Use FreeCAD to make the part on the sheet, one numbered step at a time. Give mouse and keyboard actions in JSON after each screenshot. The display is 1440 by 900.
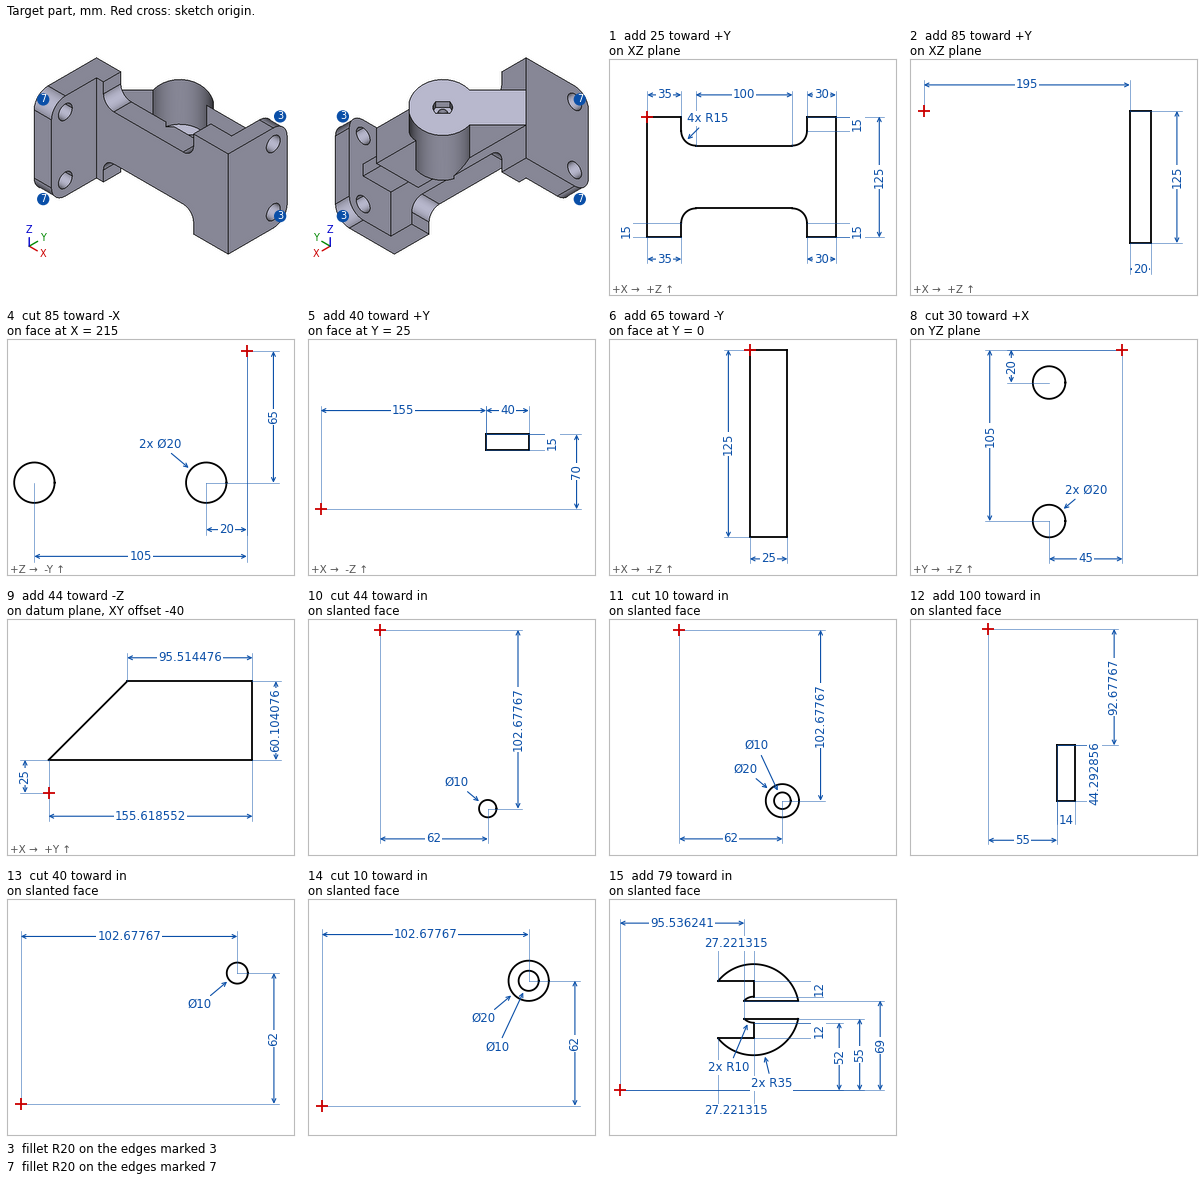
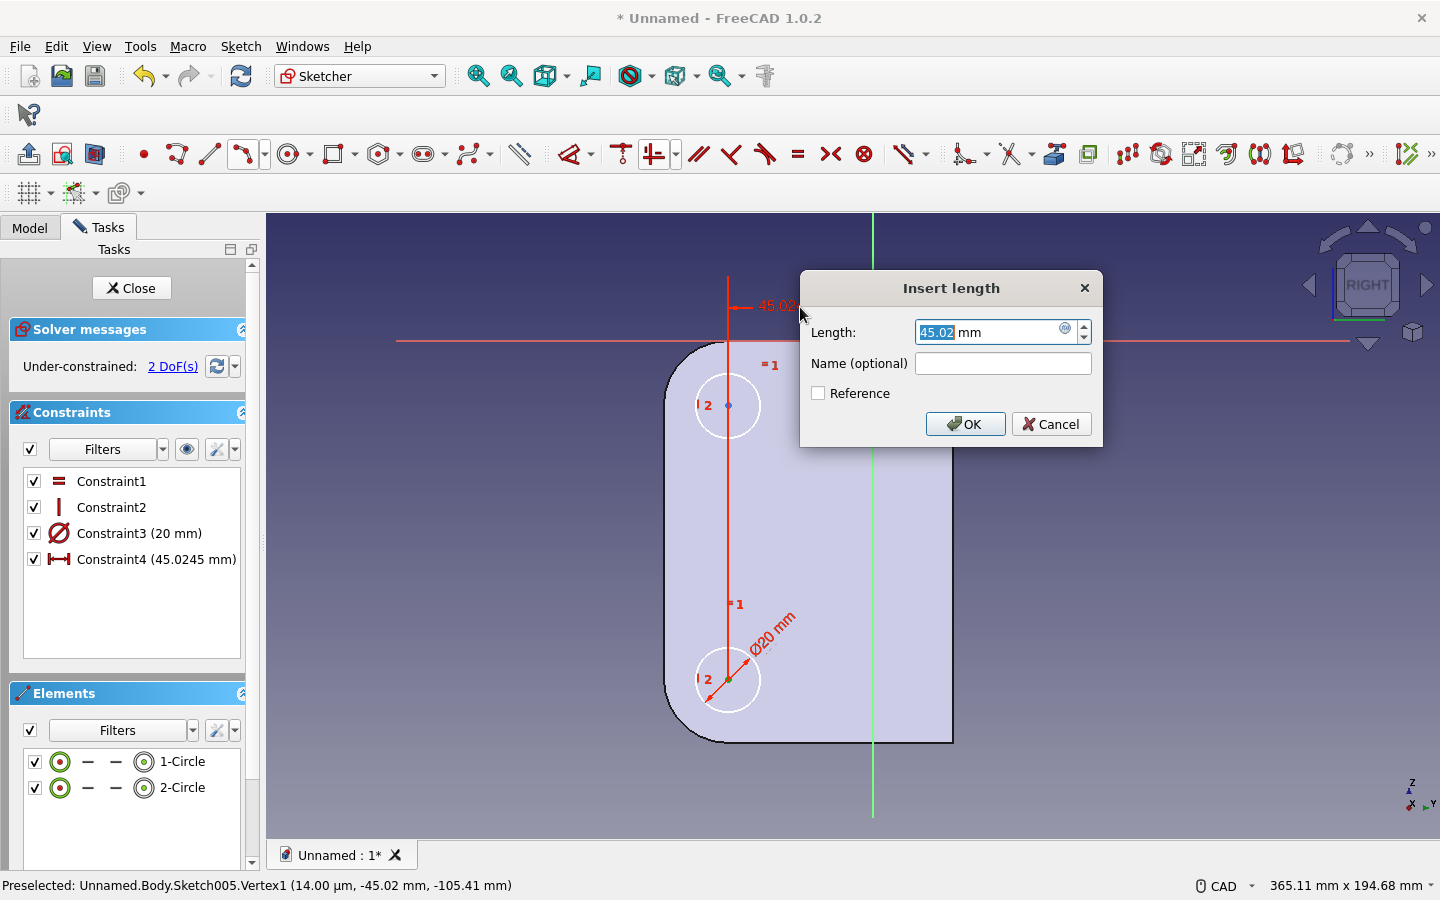
{"action": "type", "text": "45"}
{"action": "key", "text": "Return"}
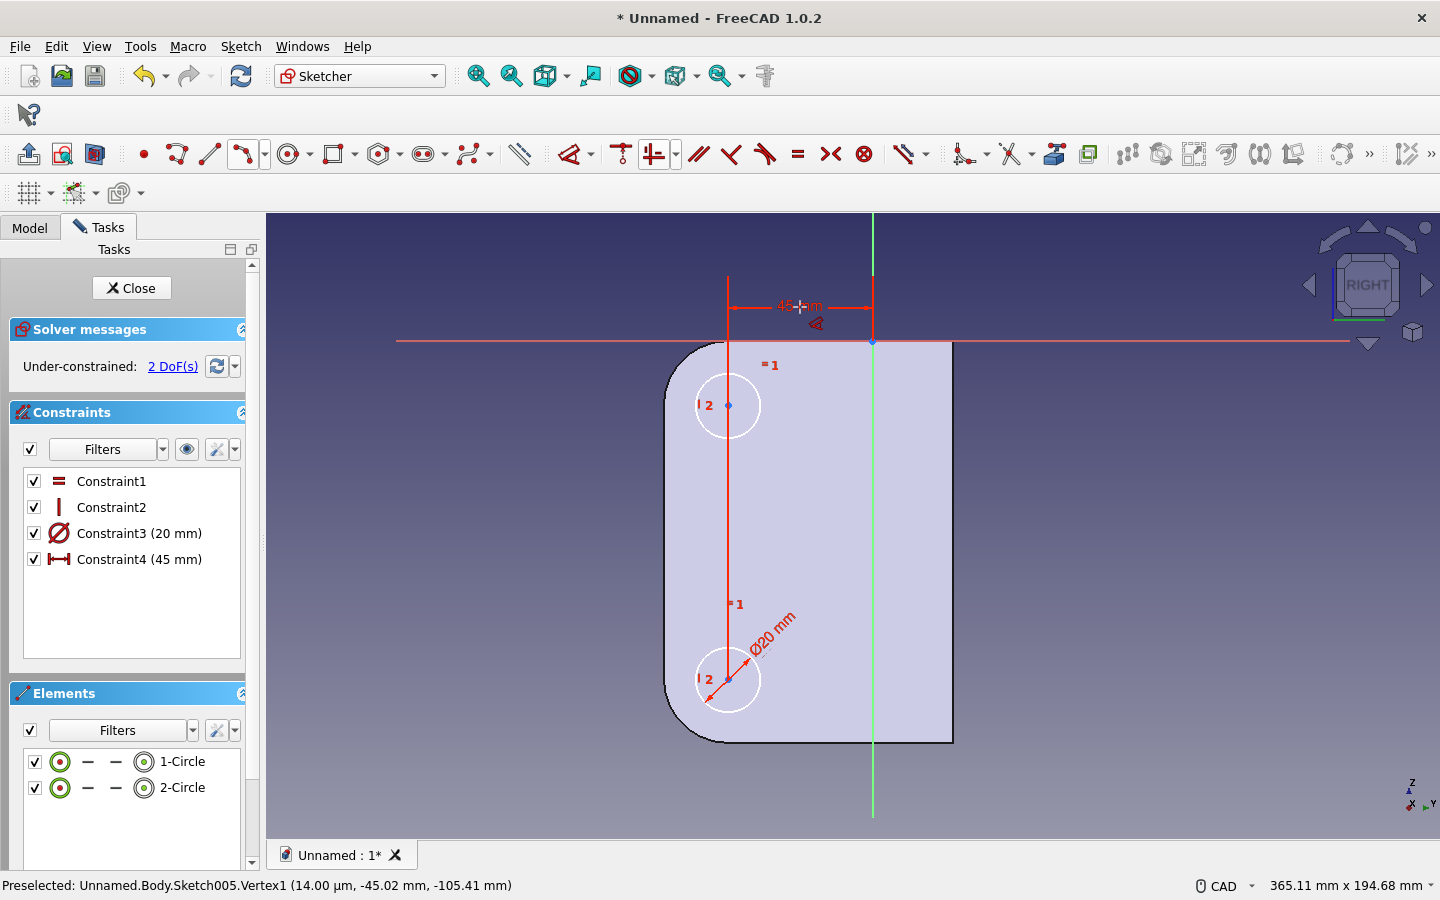
{"action": "left_click", "coordinate": [728, 406]}
{"action": "left_click", "coordinate": [907, 374]}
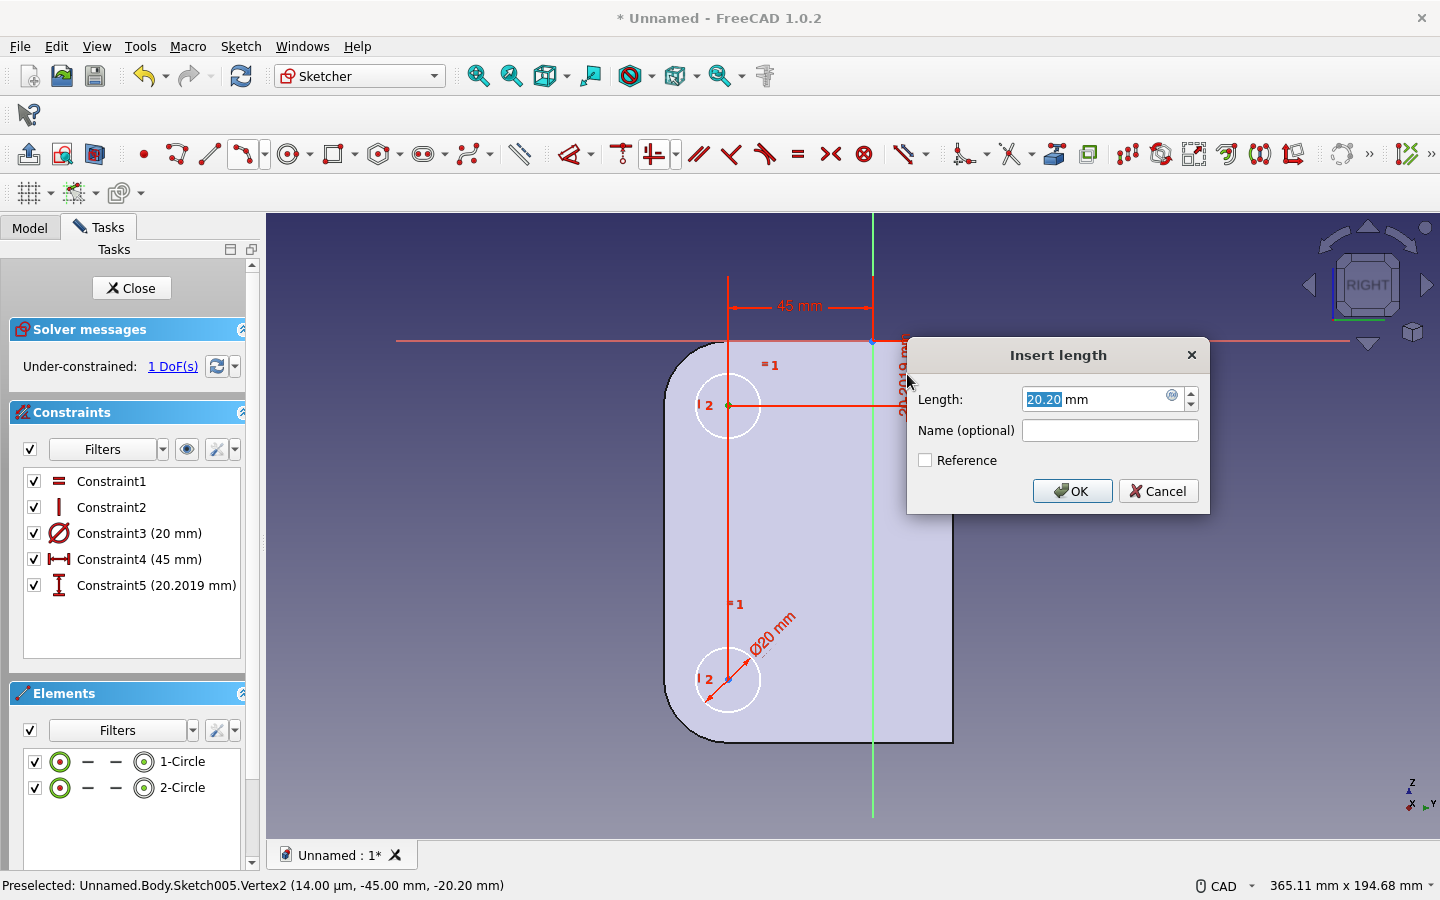
{"action": "type", "text": "20"}
{"action": "key", "text": "Return"}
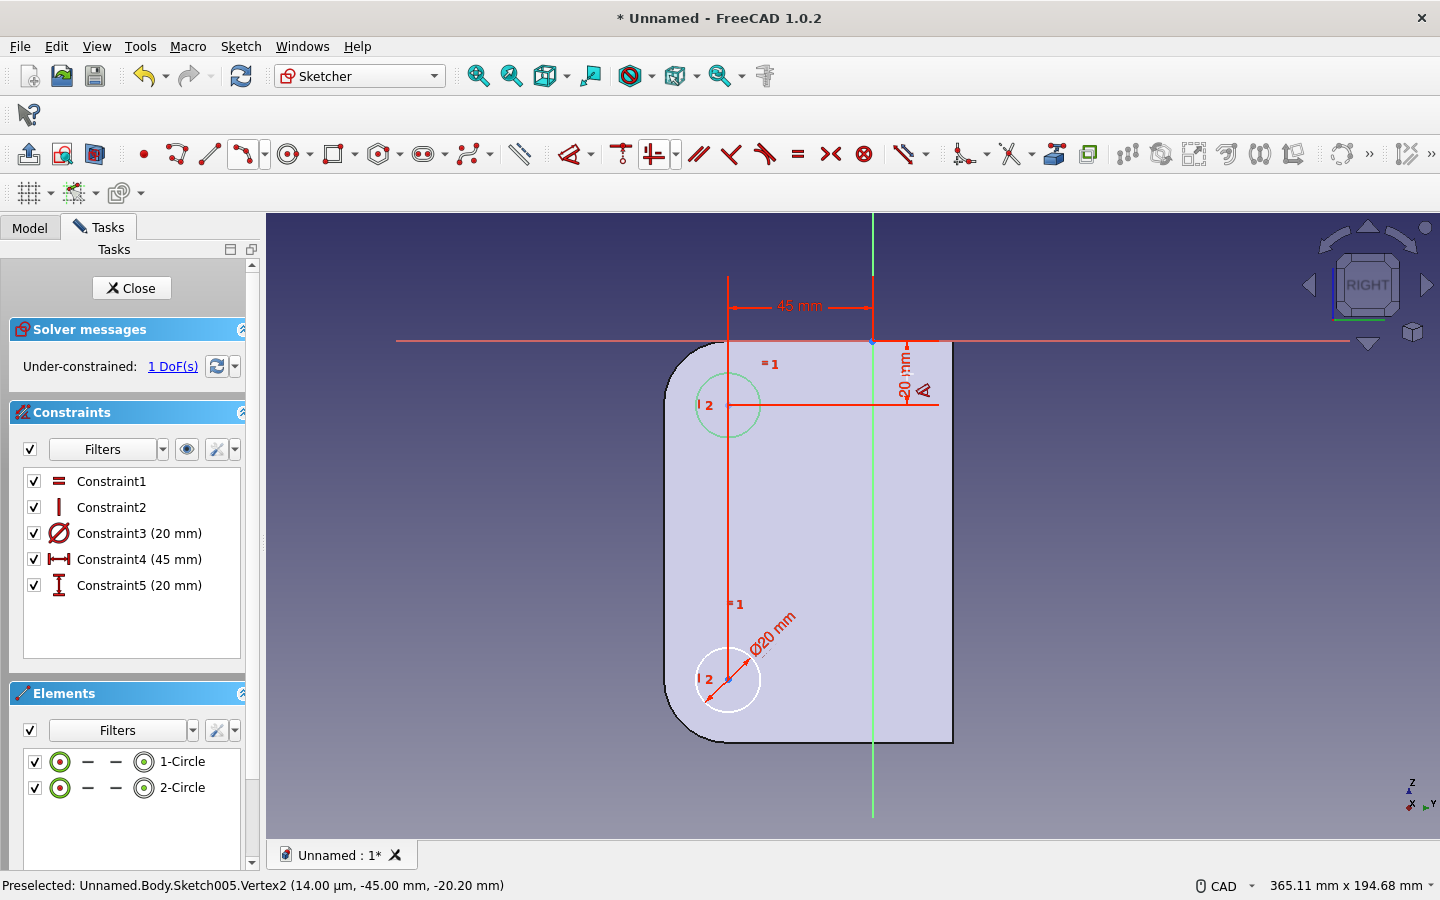
{"action": "left_click", "coordinate": [728, 680]}
{"action": "left_click", "coordinate": [907, 511]}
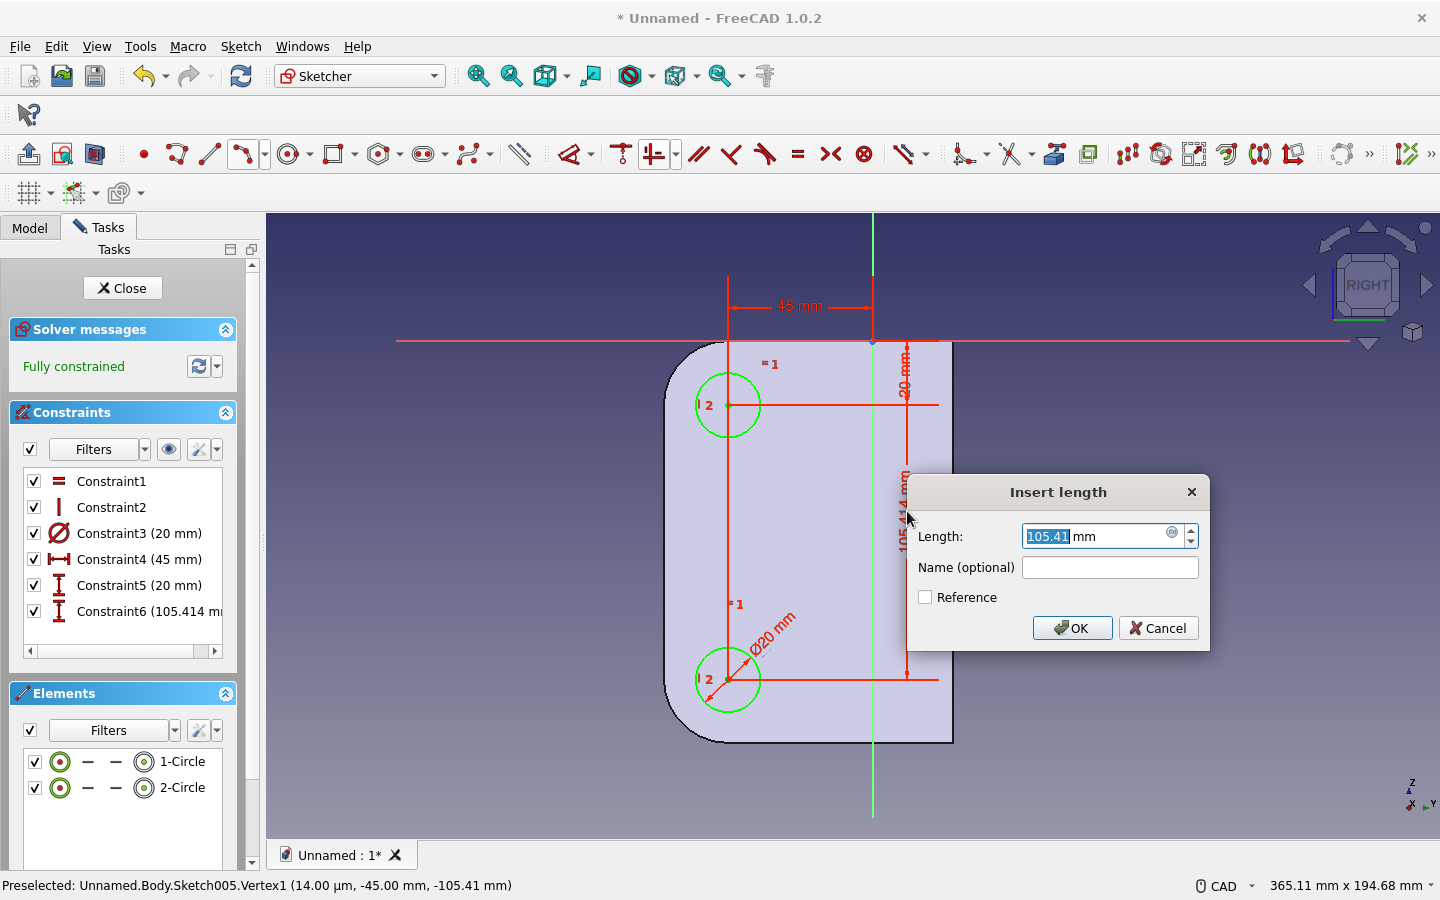
{"action": "type", "text": "105"}
{"action": "key", "text": "Return"}
{"action": "key", "text": "Escape"}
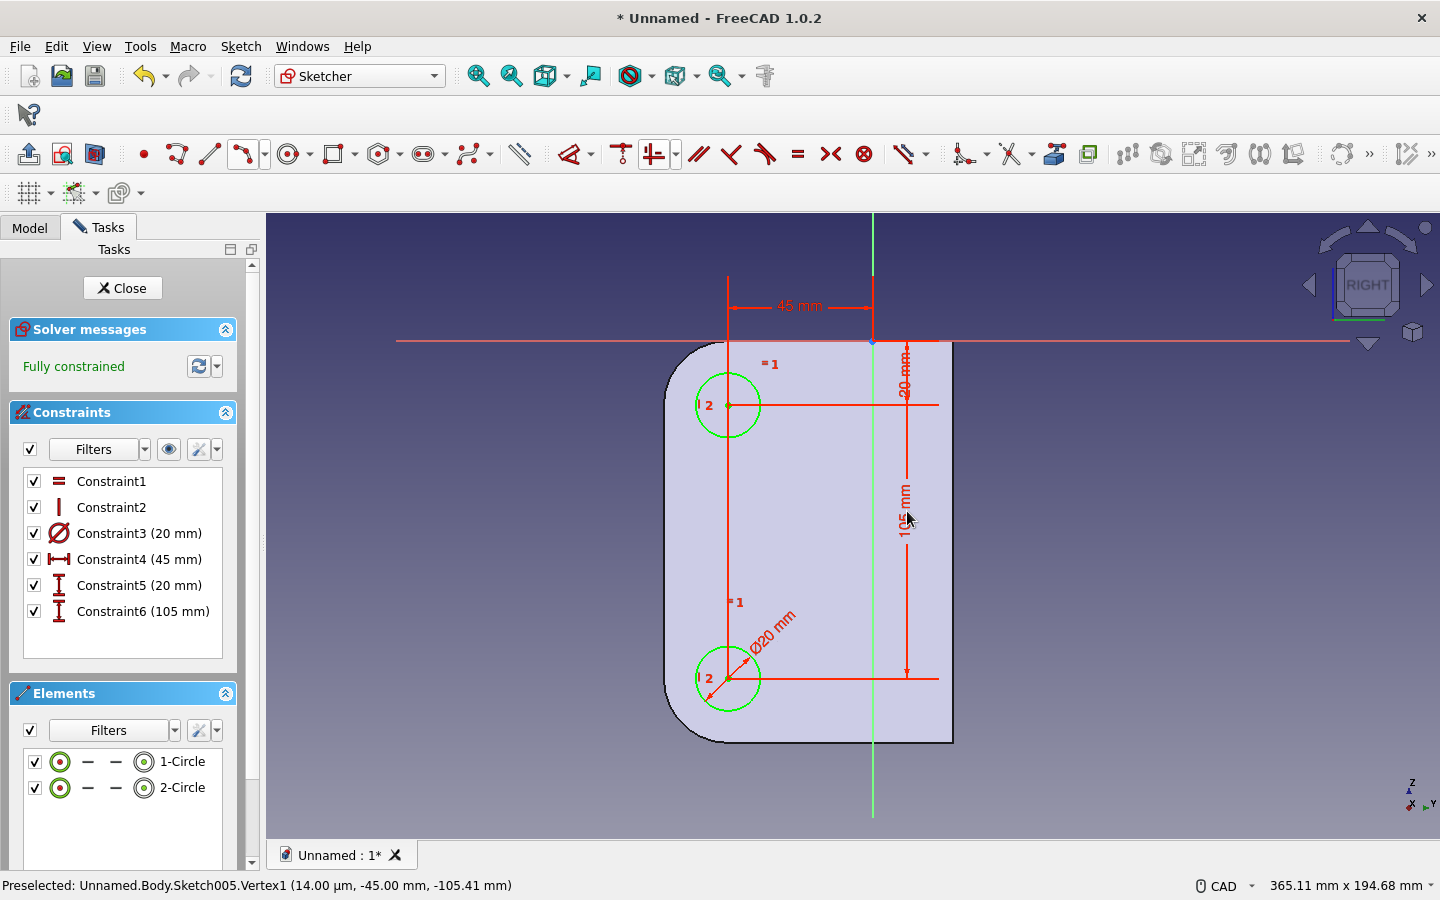
{"action": "left_click", "coordinate": [123, 288]}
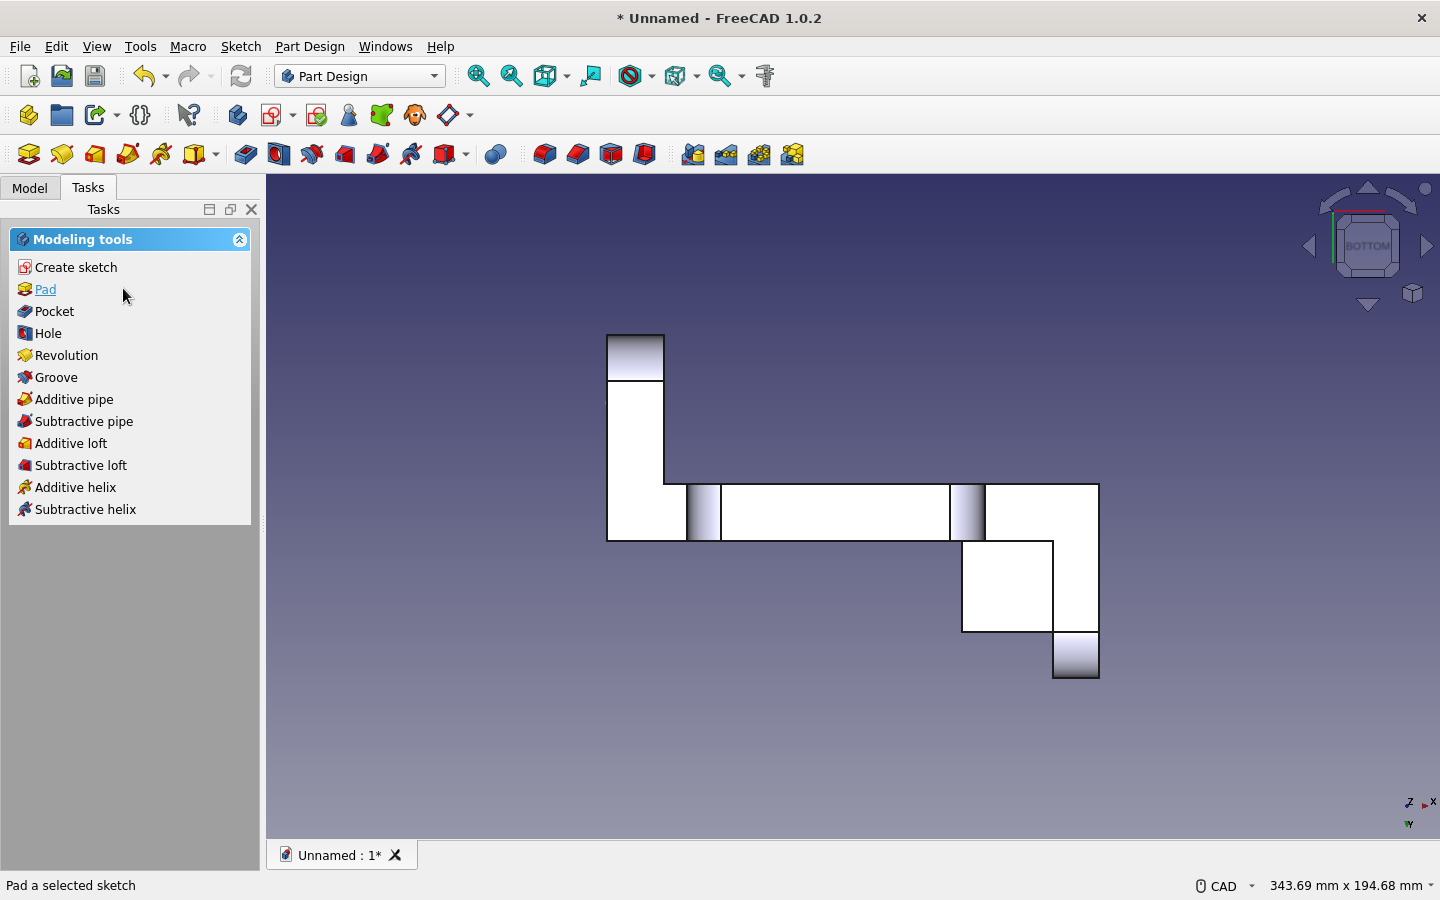
{"action": "left_click", "coordinate": [246, 154]}